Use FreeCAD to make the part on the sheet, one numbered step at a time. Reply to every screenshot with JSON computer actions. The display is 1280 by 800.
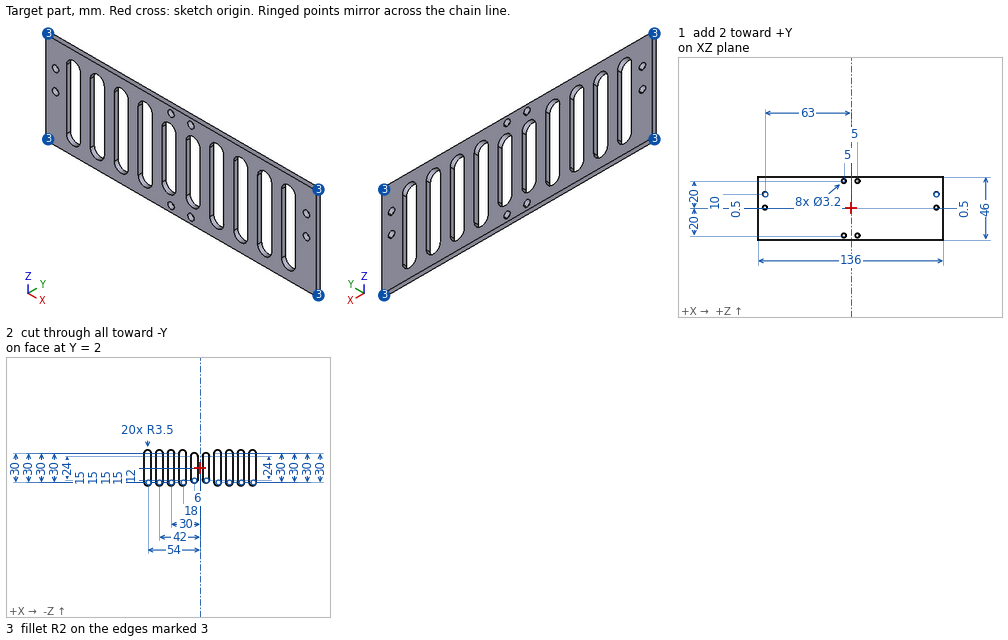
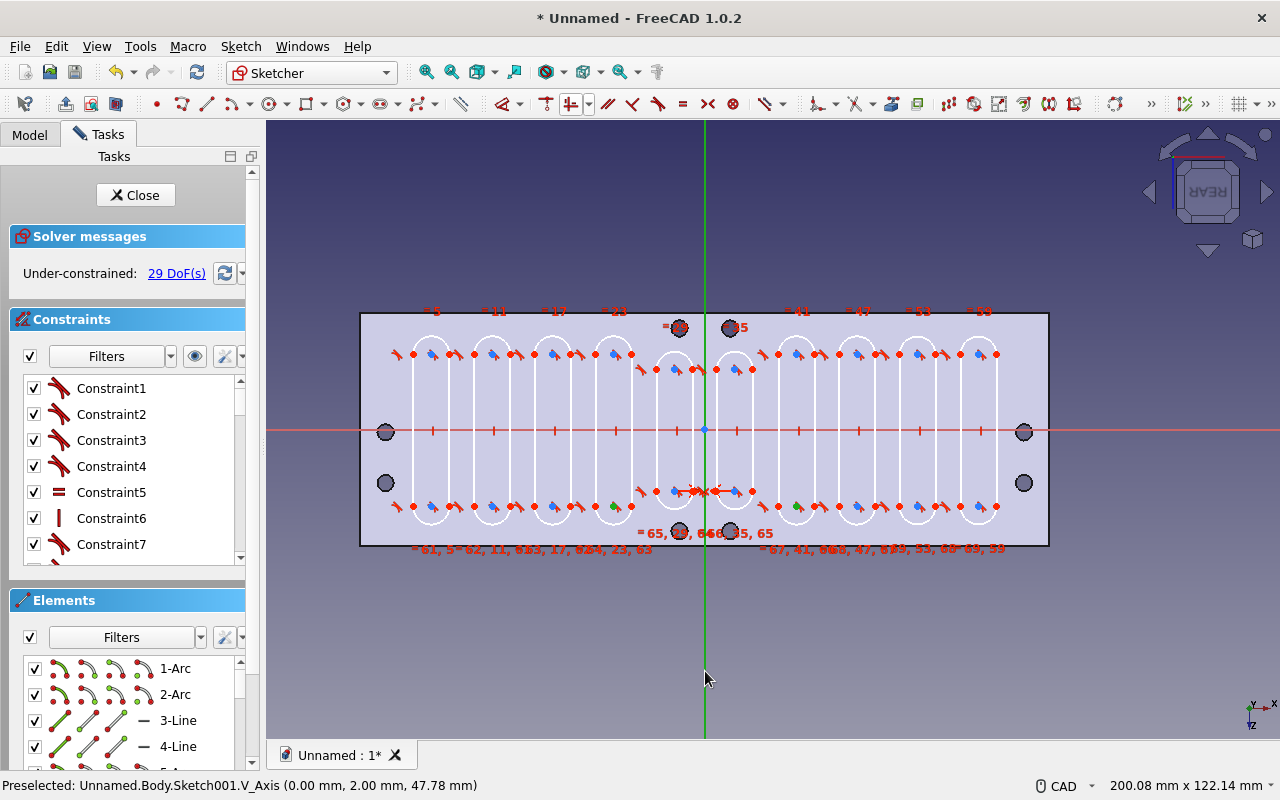
{"action": "left_click", "coordinate": [708, 104]}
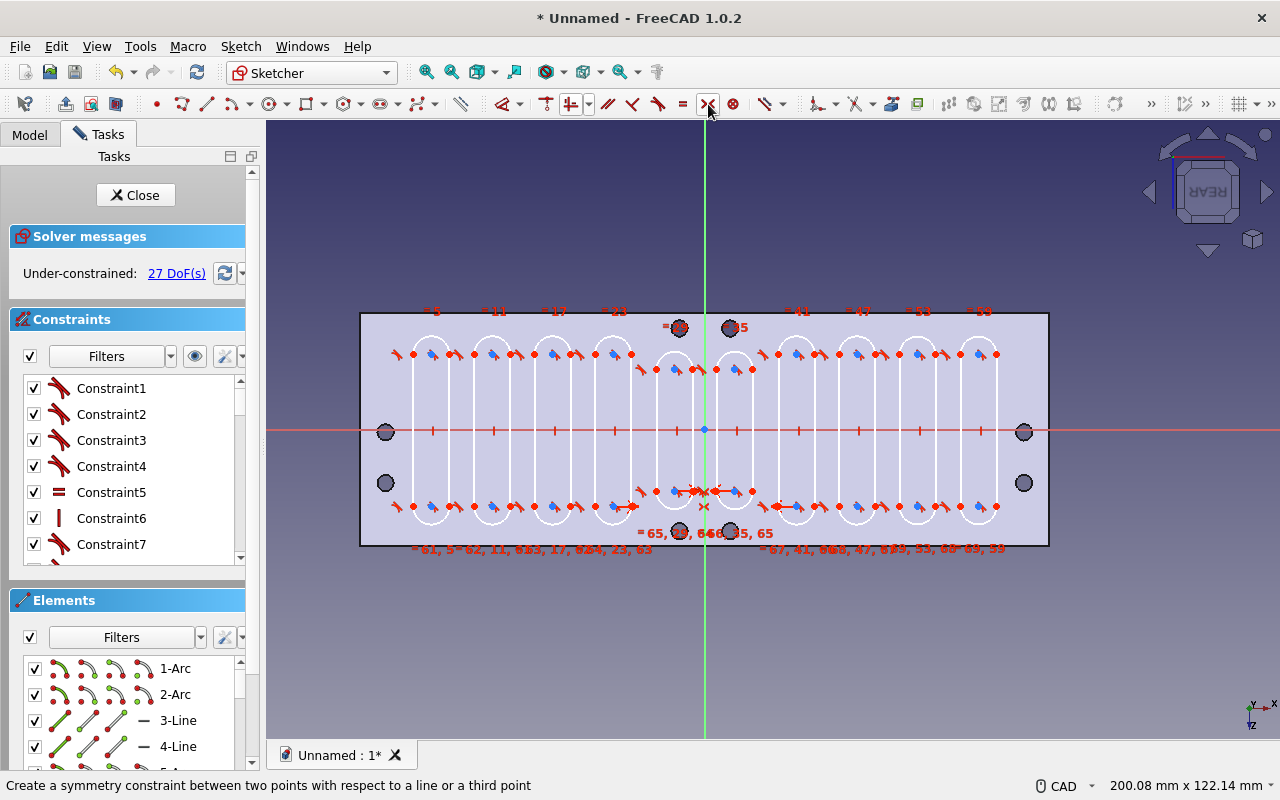
{"action": "left_click", "coordinate": [553, 507]}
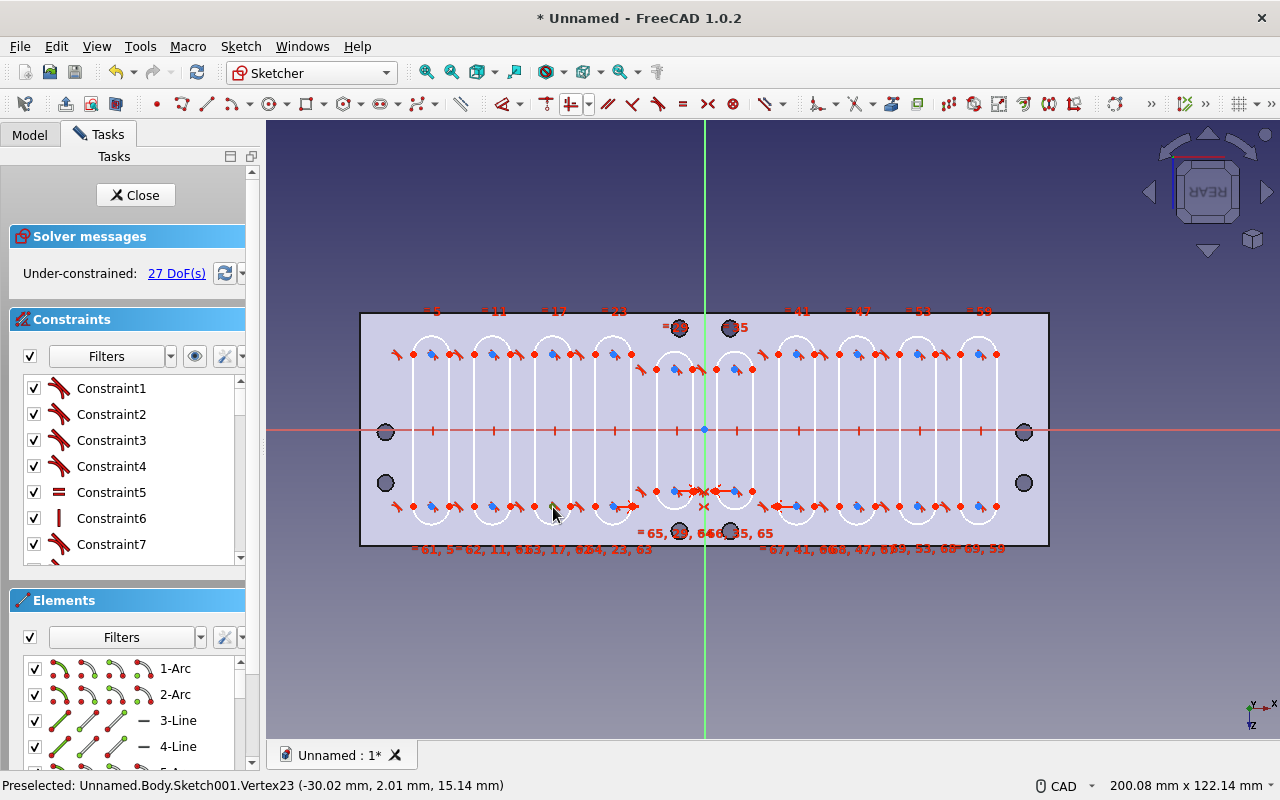
{"action": "left_click", "coordinate": [857, 507]}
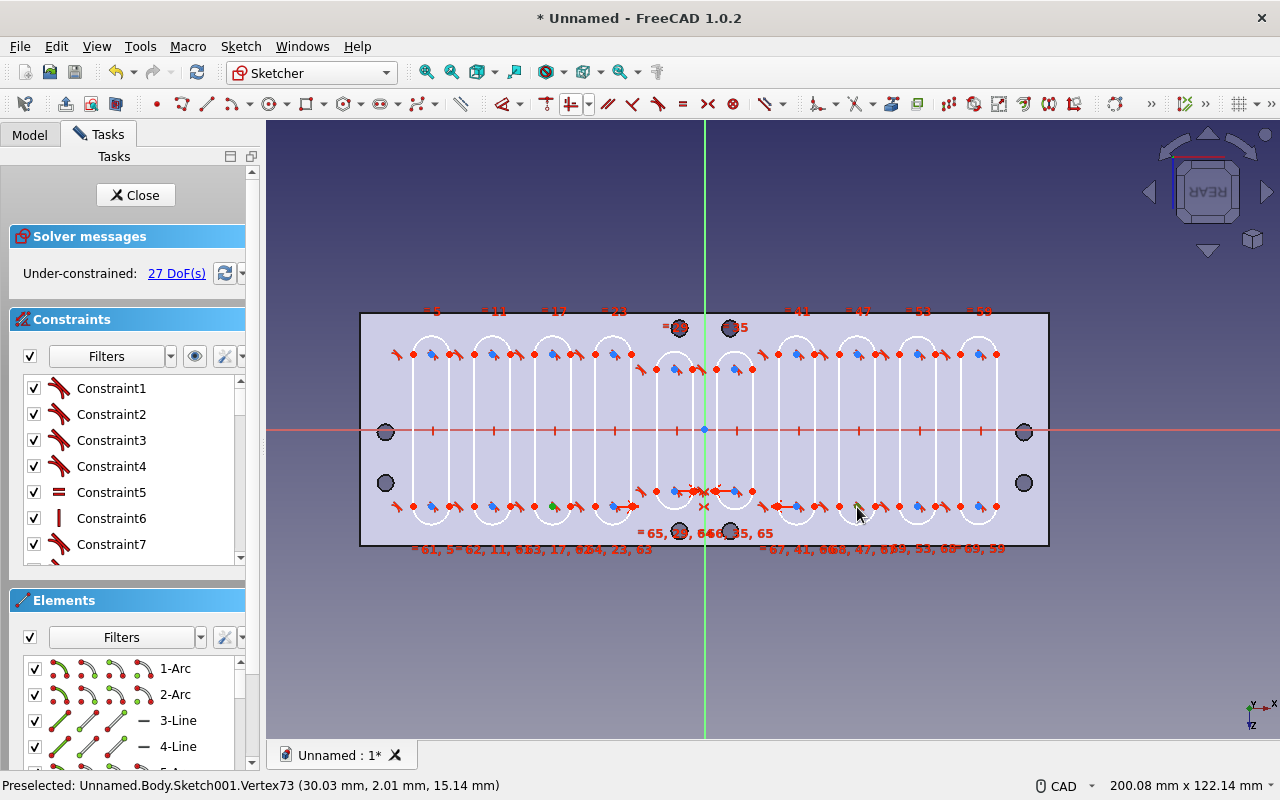
{"action": "left_click", "coordinate": [705, 671]}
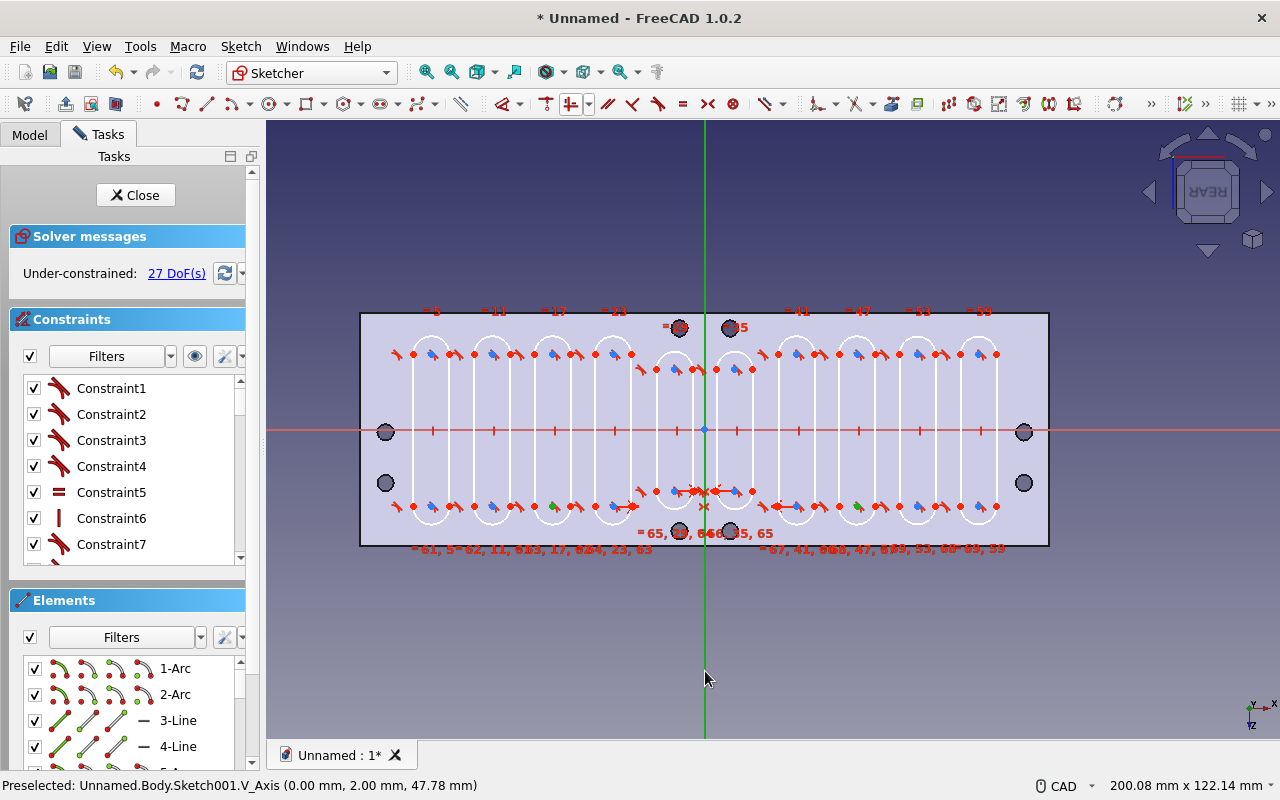
{"action": "left_click", "coordinate": [708, 104]}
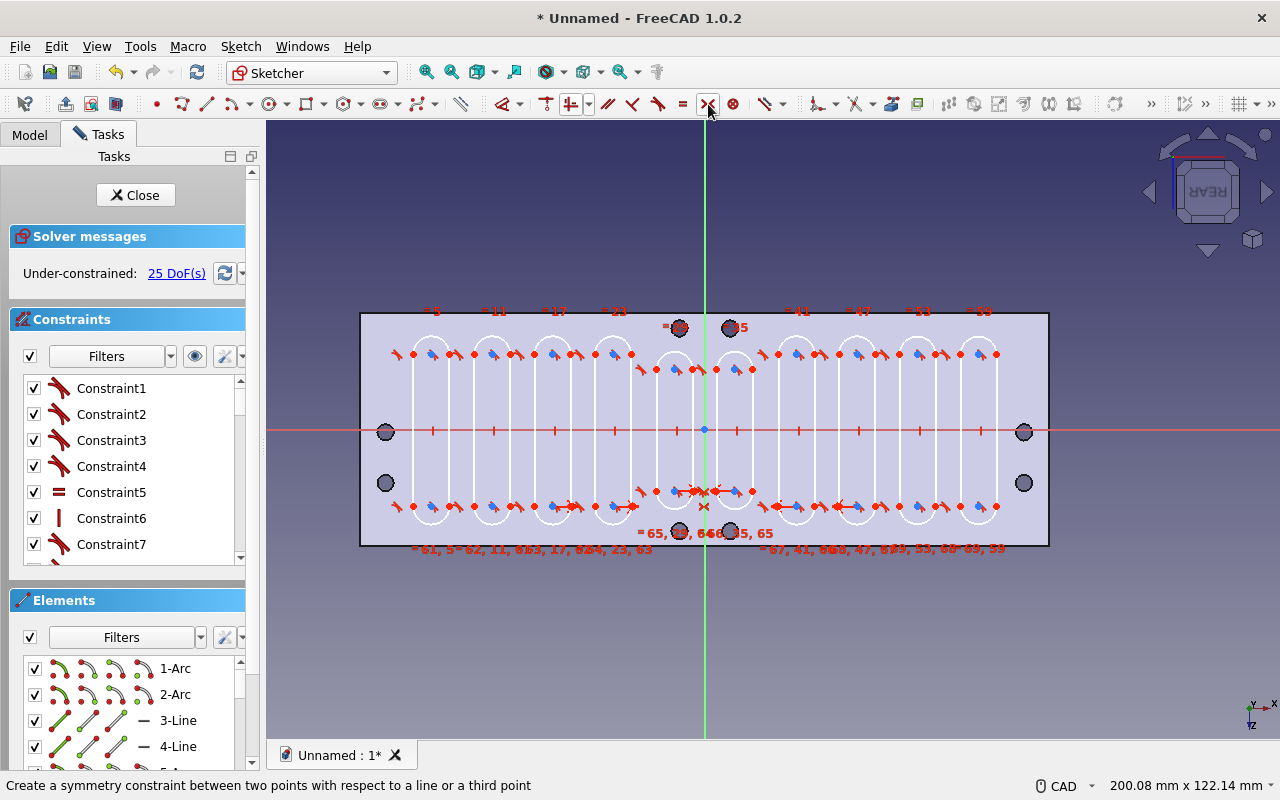
{"action": "left_click", "coordinate": [492, 507]}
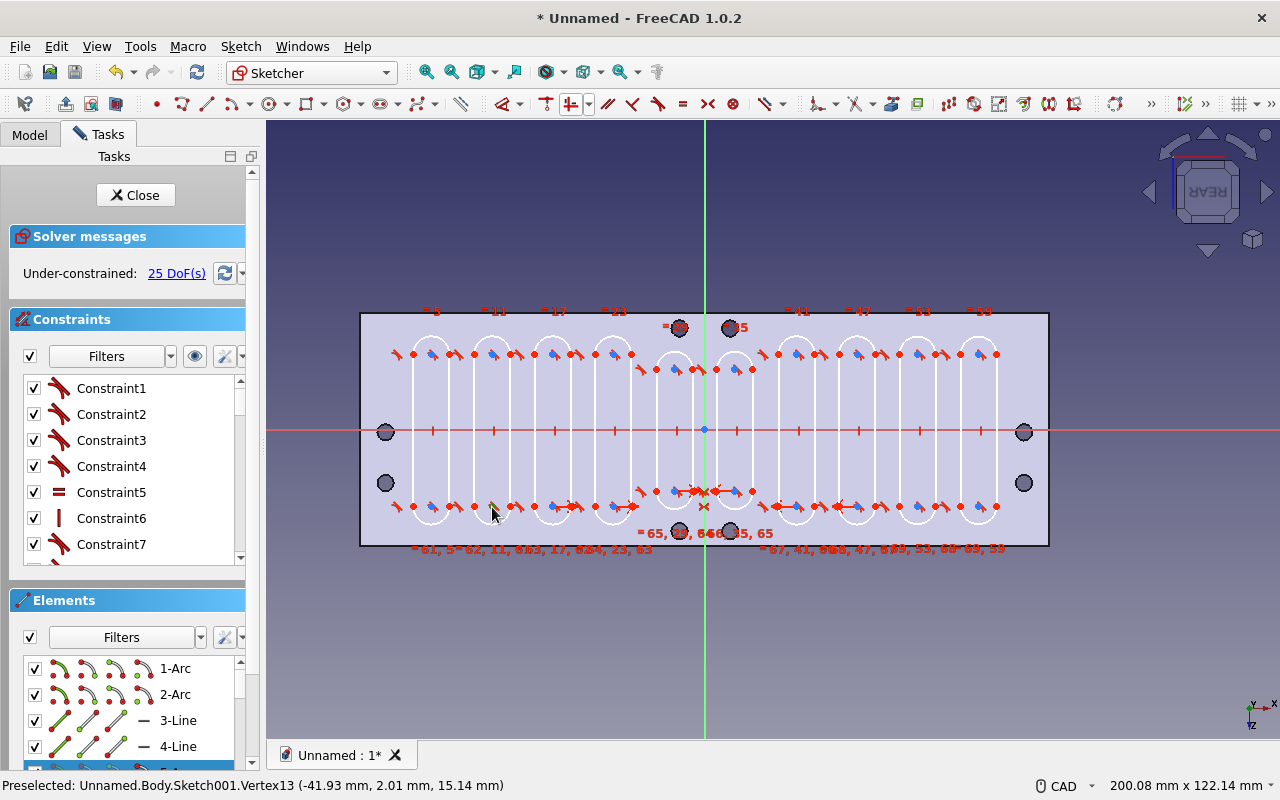
{"action": "left_click", "coordinate": [918, 506]}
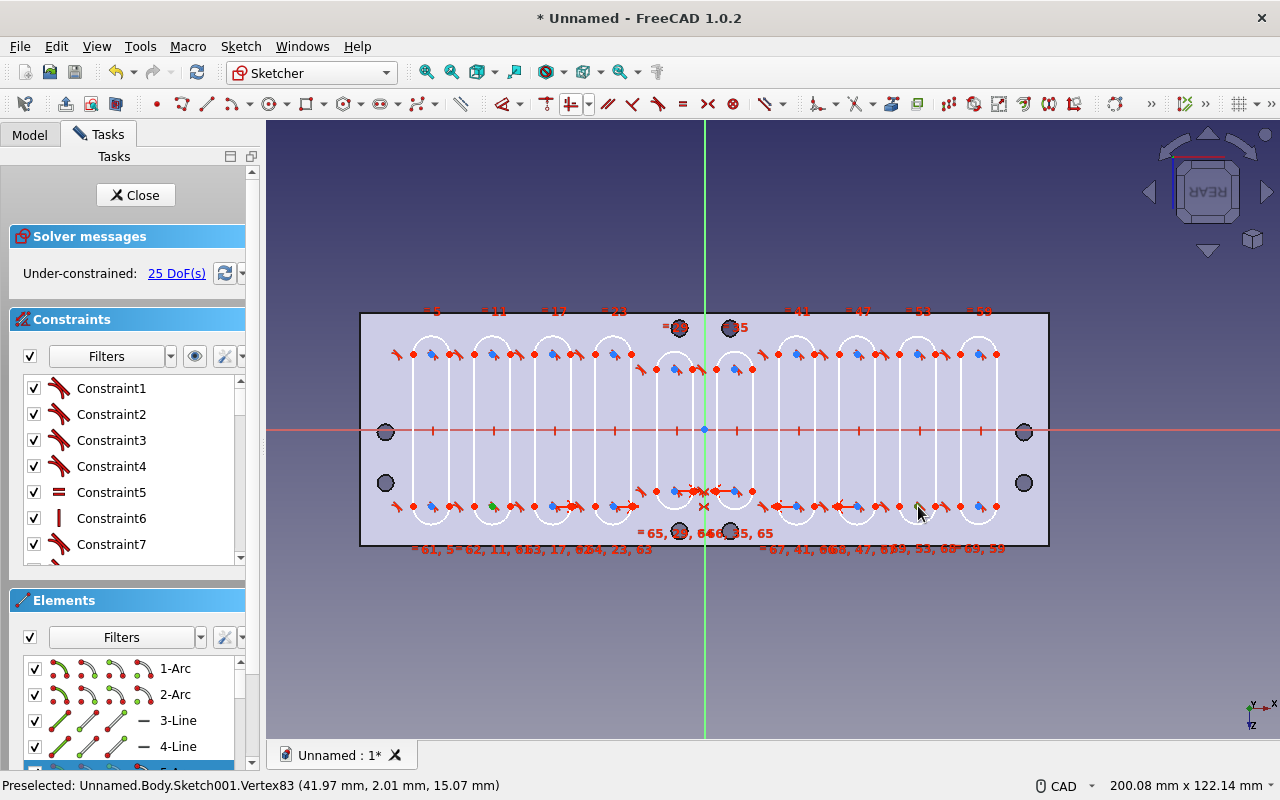
{"action": "left_click", "coordinate": [705, 671]}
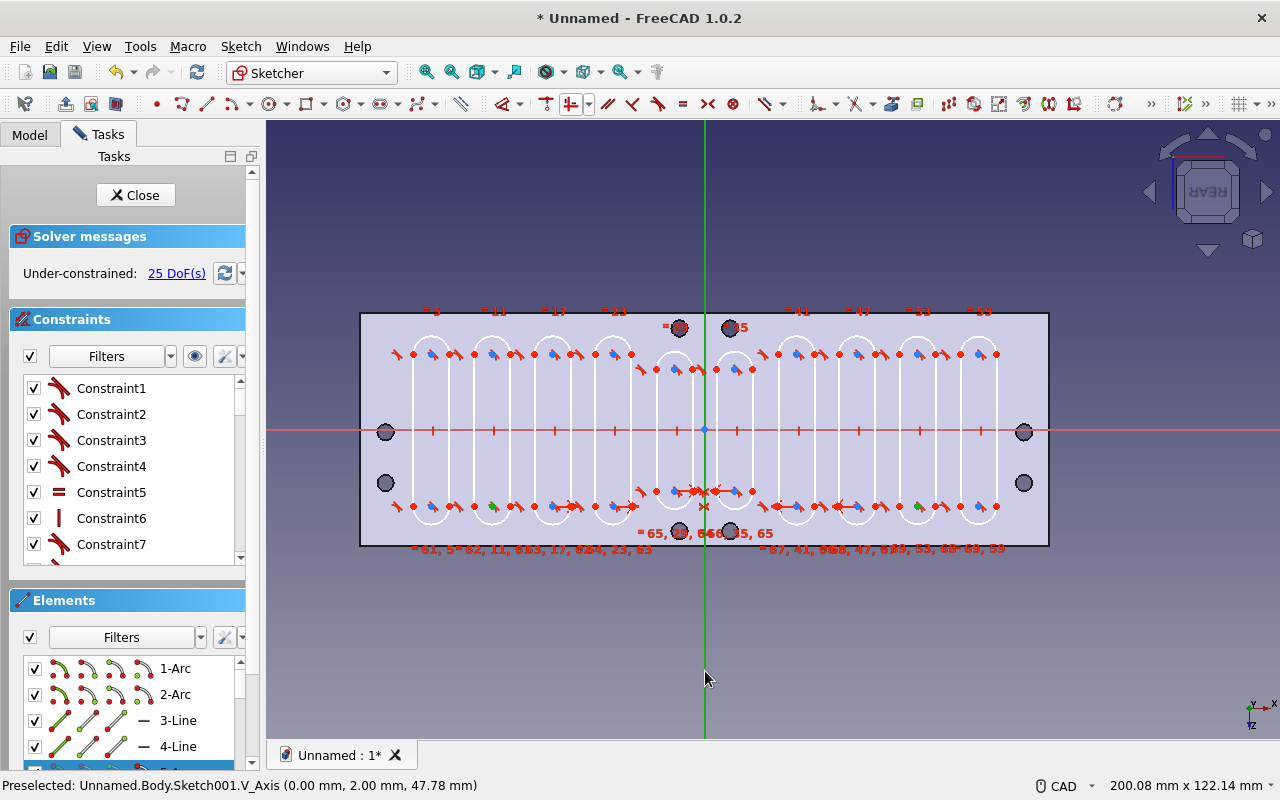
{"action": "left_click", "coordinate": [708, 104]}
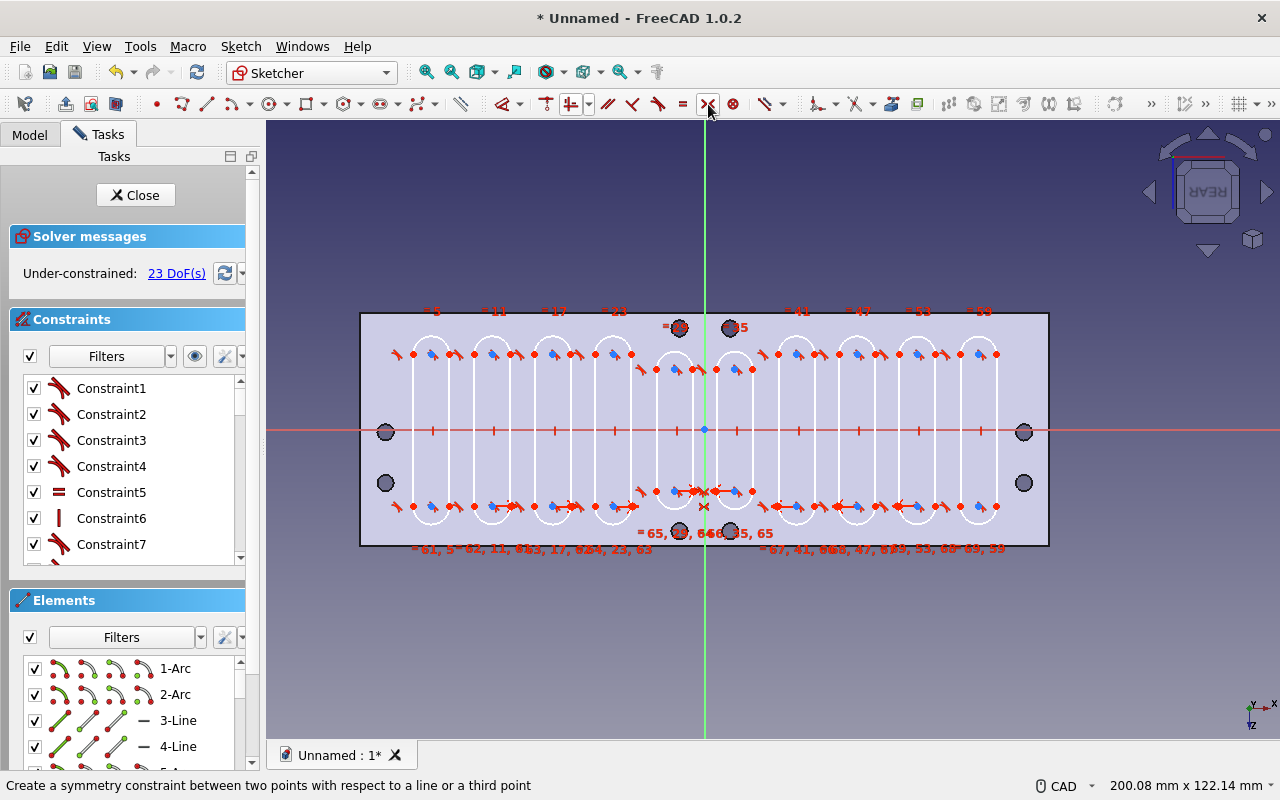
{"action": "left_click", "coordinate": [431, 507]}